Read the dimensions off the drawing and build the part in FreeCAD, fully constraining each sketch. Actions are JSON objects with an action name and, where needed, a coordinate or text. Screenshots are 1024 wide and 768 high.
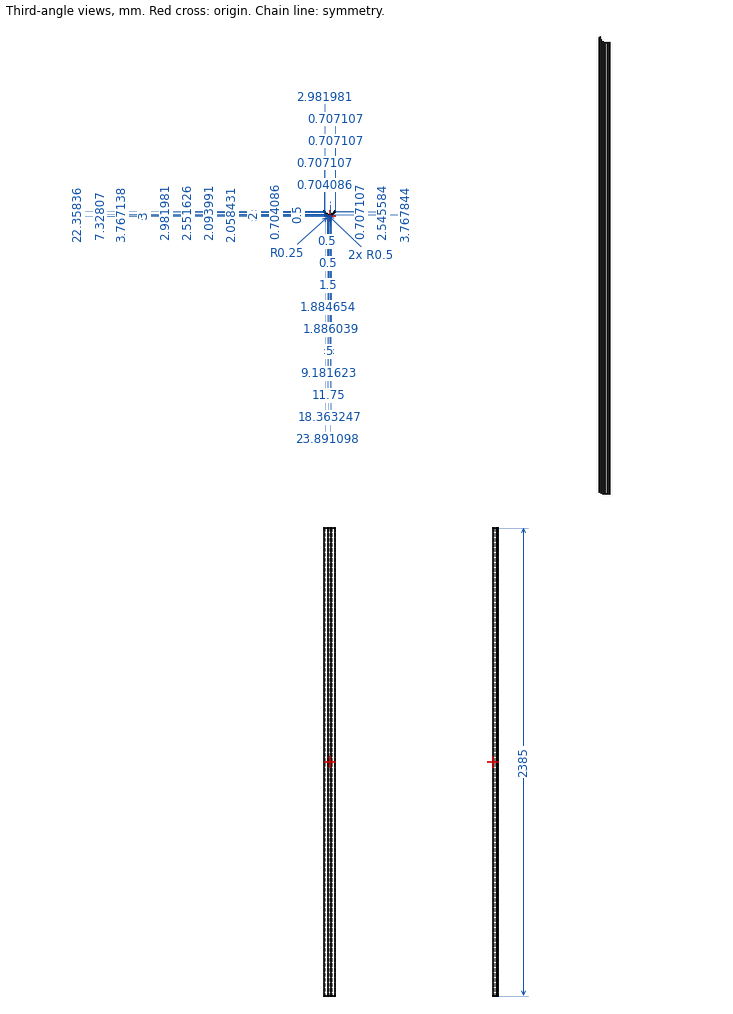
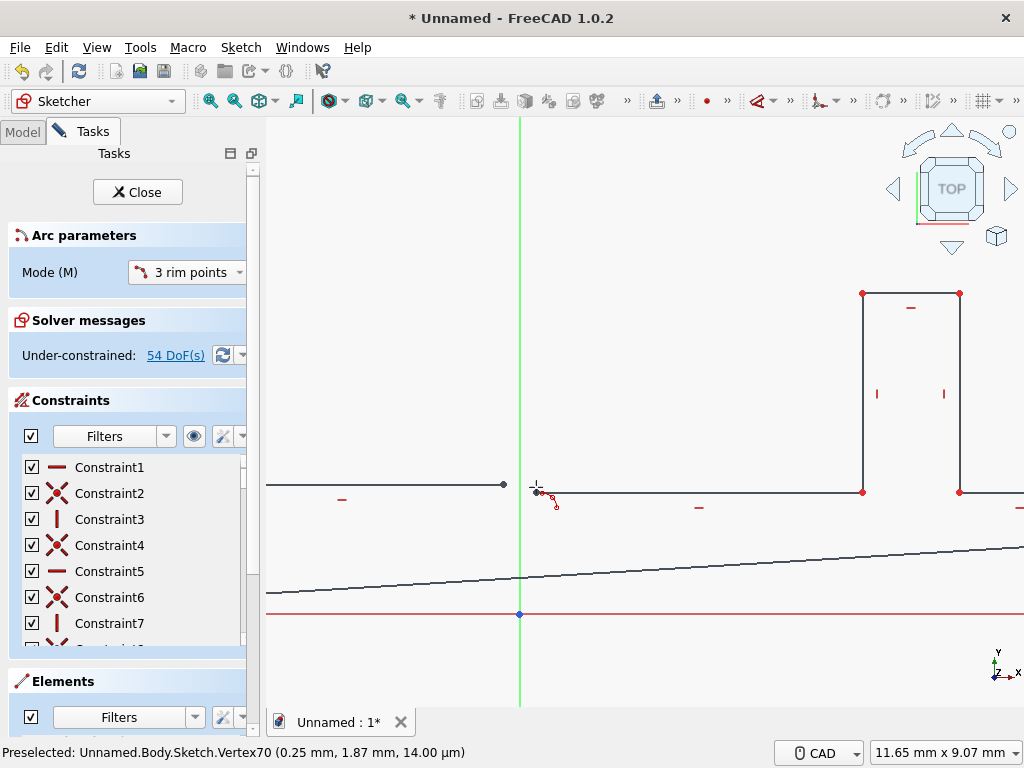
{"action": "scroll", "coordinate": [584, 477], "scroll_direction": "down", "scroll_amount": 11}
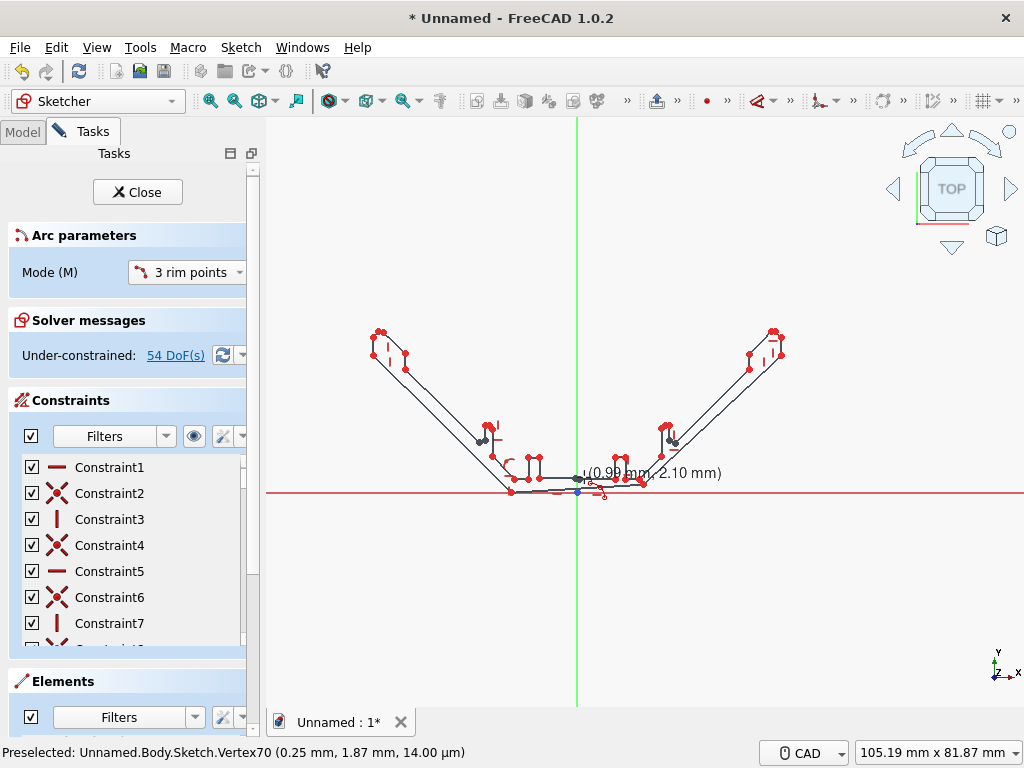
{"action": "scroll", "coordinate": [485, 440], "scroll_direction": "up", "scroll_amount": 5}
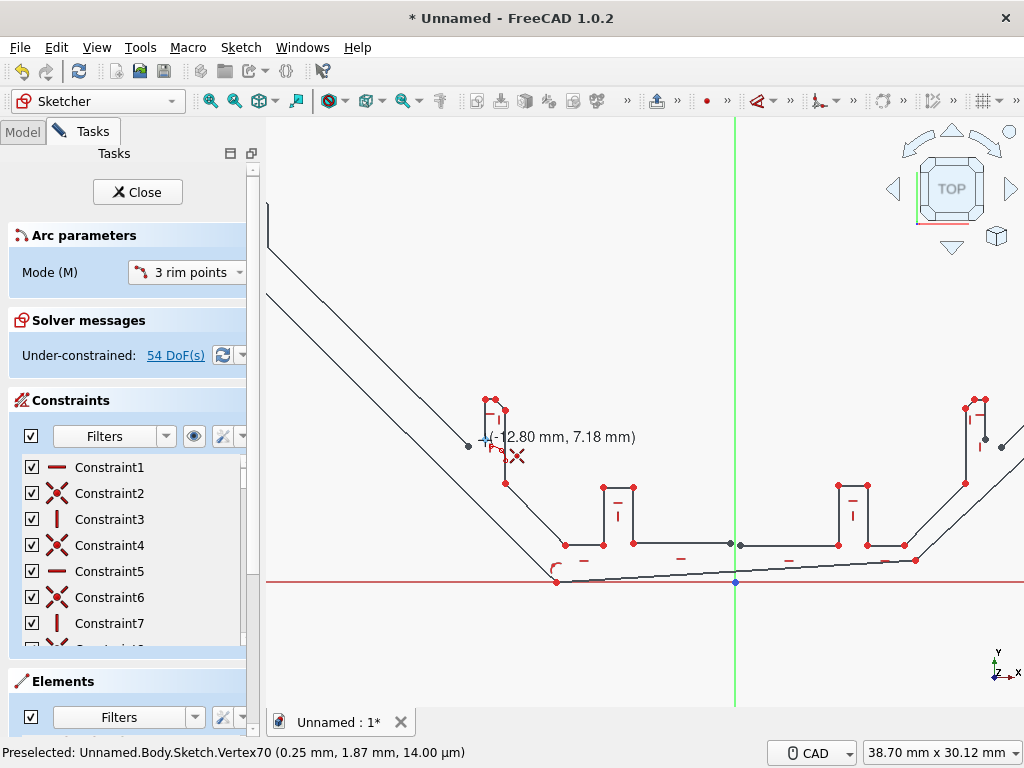
{"action": "left_click", "coordinate": [485, 440]}
{"action": "left_click", "coordinate": [469, 446]}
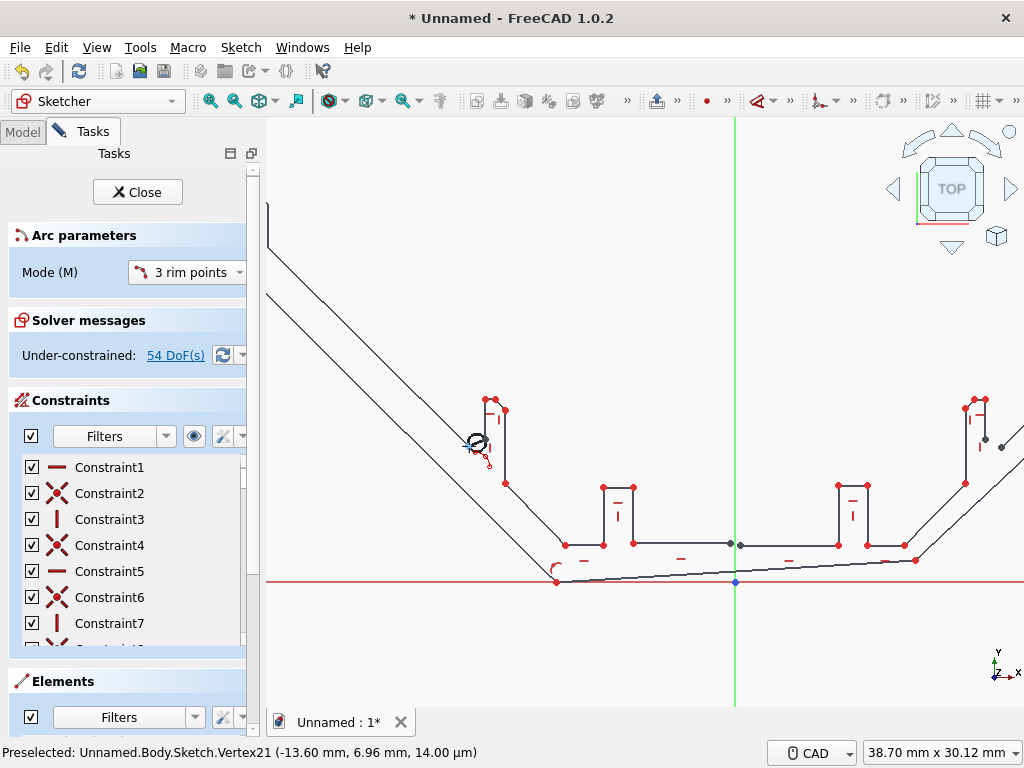
{"action": "scroll", "coordinate": [479, 448], "scroll_direction": "up", "scroll_amount": 5}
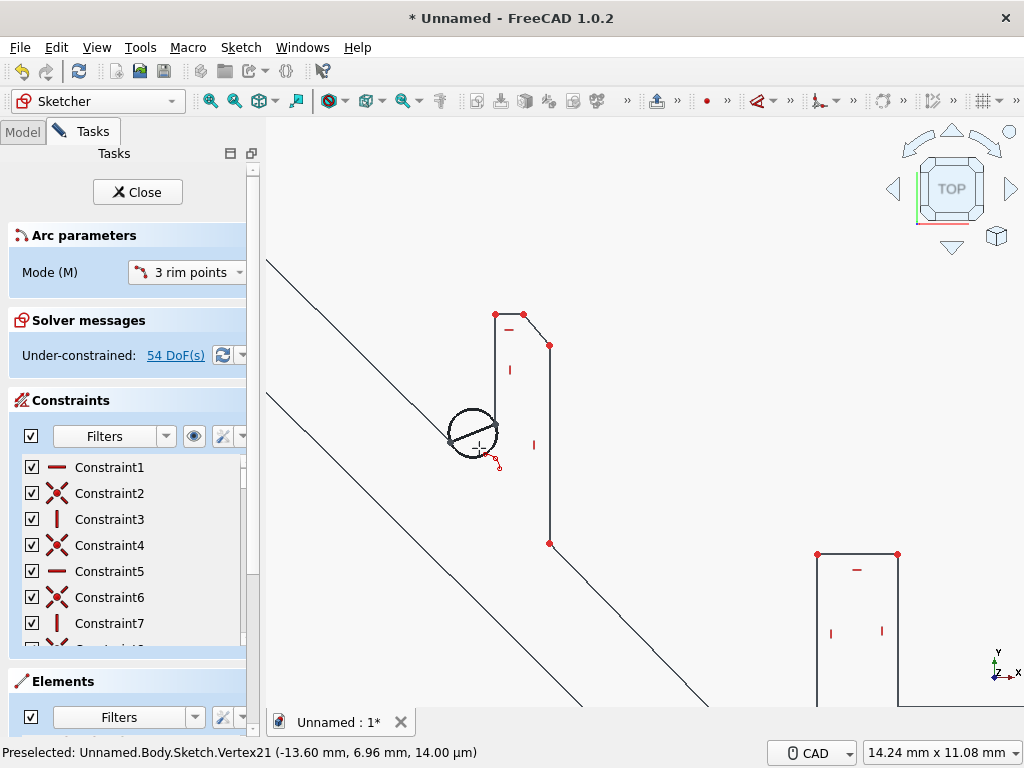
{"action": "left_click", "coordinate": [480, 447]}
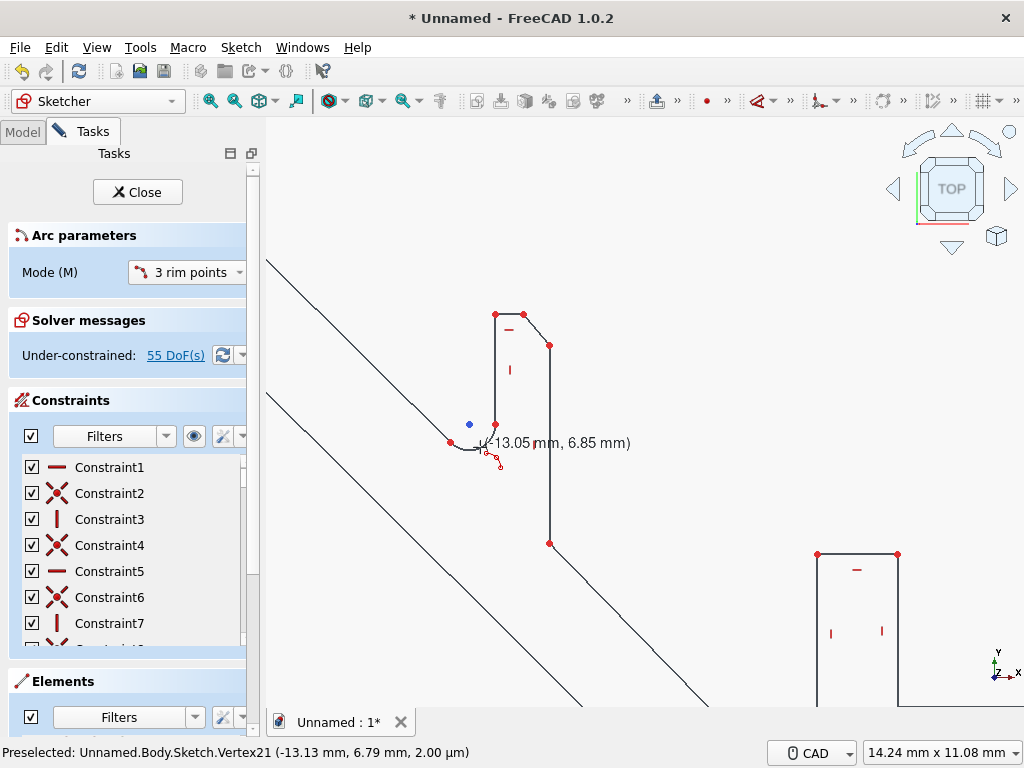
{"action": "scroll", "coordinate": [483, 442], "scroll_direction": "down", "scroll_amount": 10}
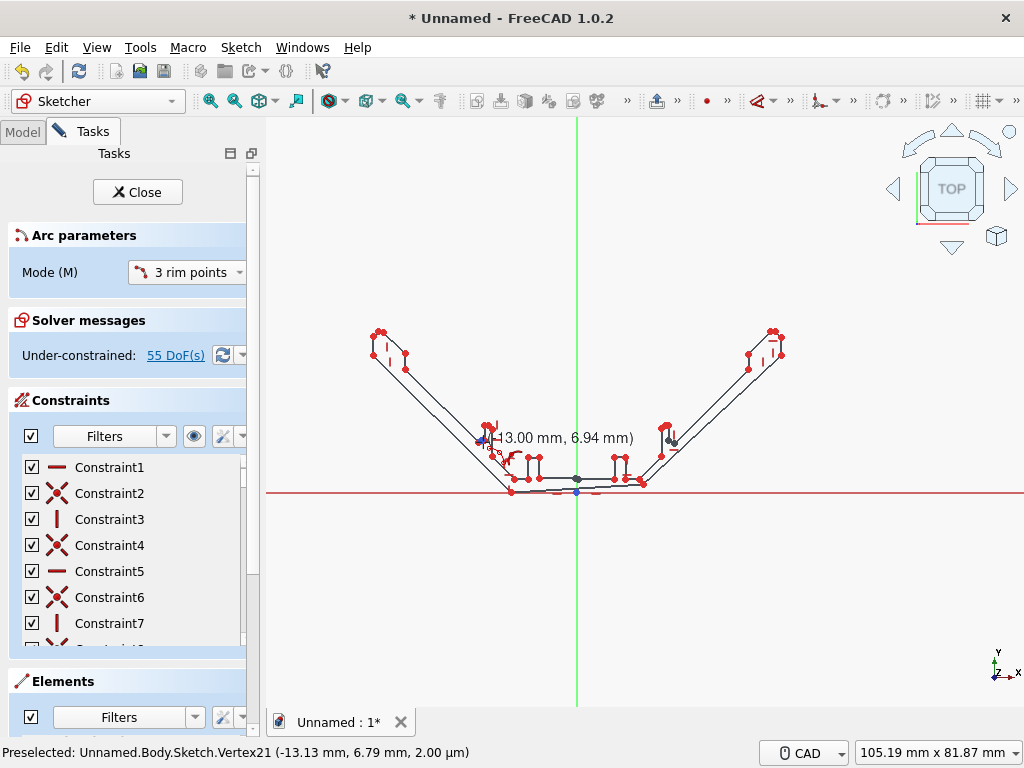
{"action": "scroll", "coordinate": [675, 442], "scroll_direction": "up", "scroll_amount": 5}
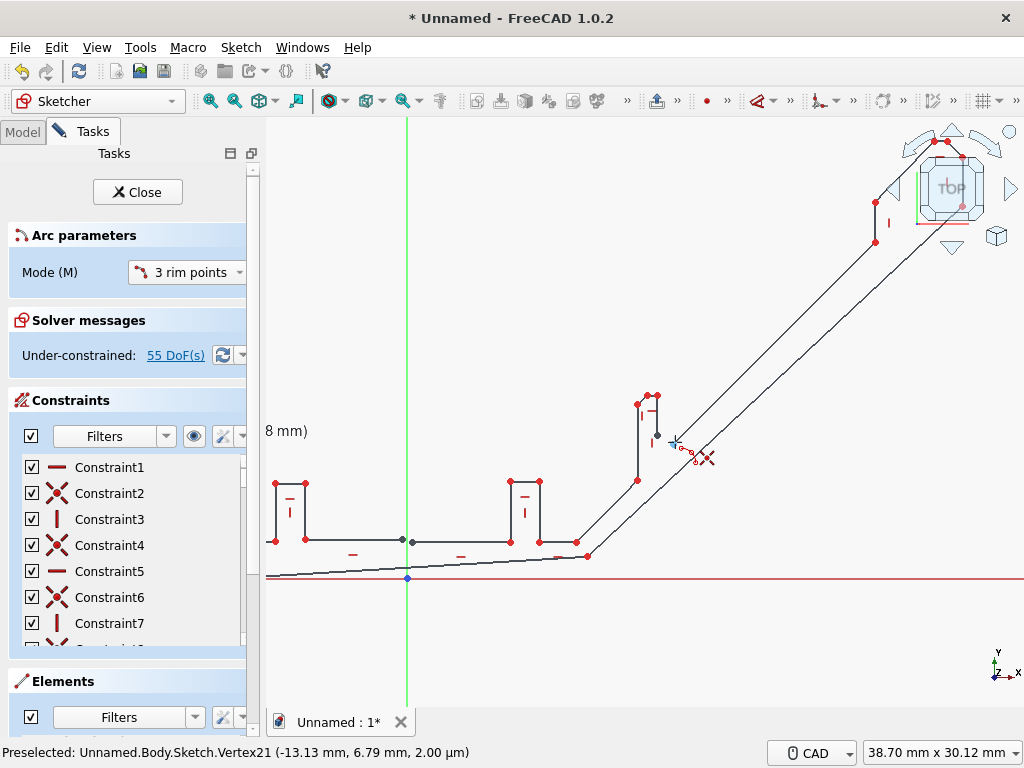
{"action": "left_click", "coordinate": [674, 444]}
{"action": "left_click", "coordinate": [657, 436]}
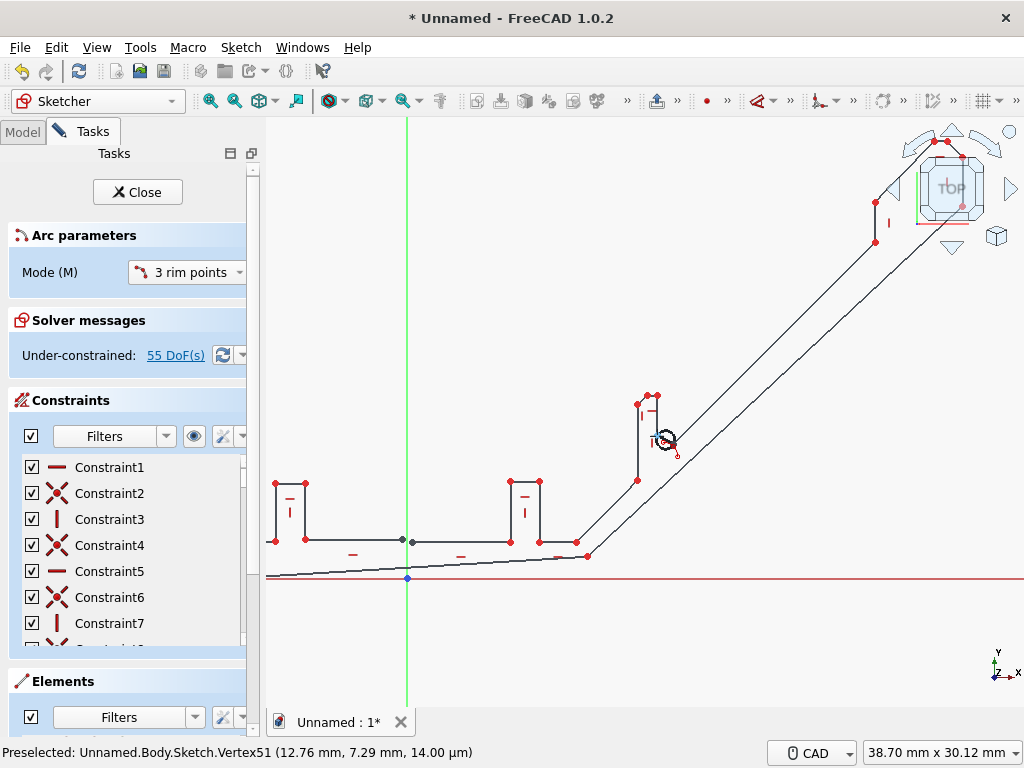
{"action": "scroll", "coordinate": [663, 444], "scroll_direction": "up", "scroll_amount": 5}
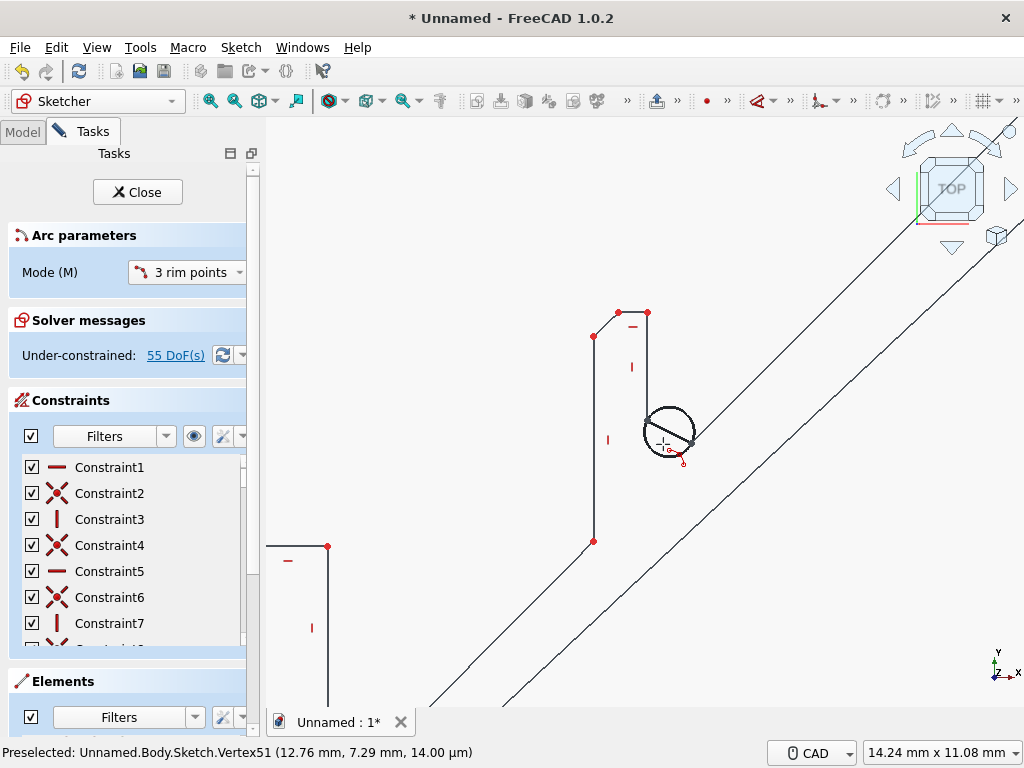
{"action": "left_click", "coordinate": [663, 443]}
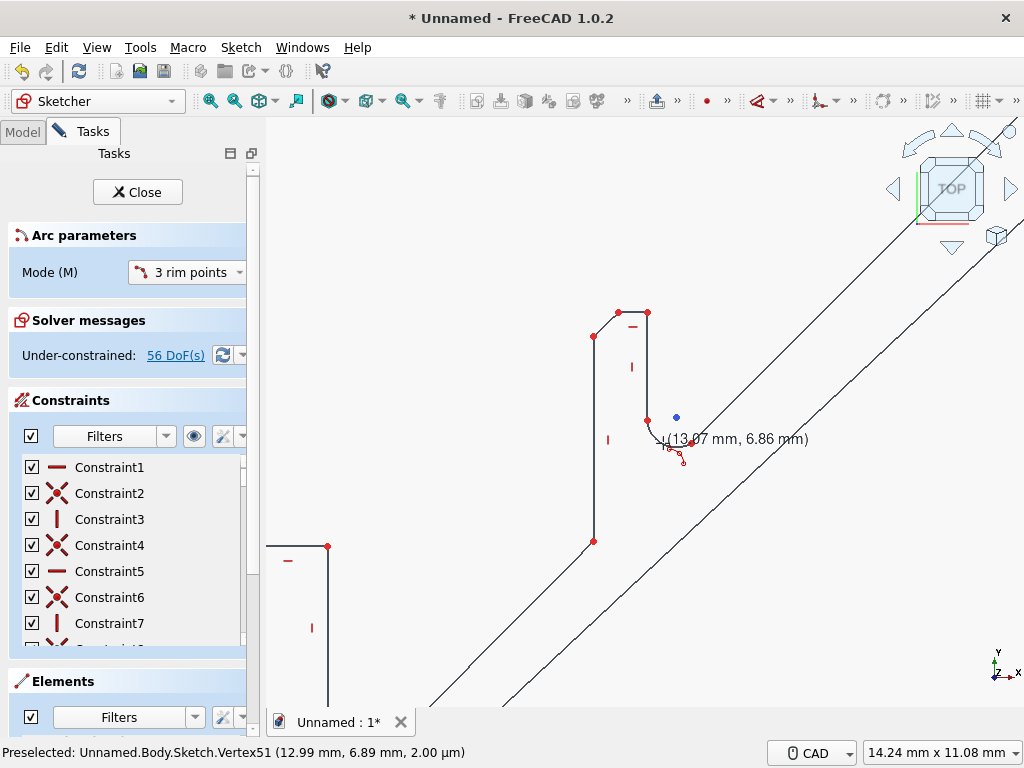
{"action": "scroll", "coordinate": [672, 443], "scroll_direction": "down", "scroll_amount": 10}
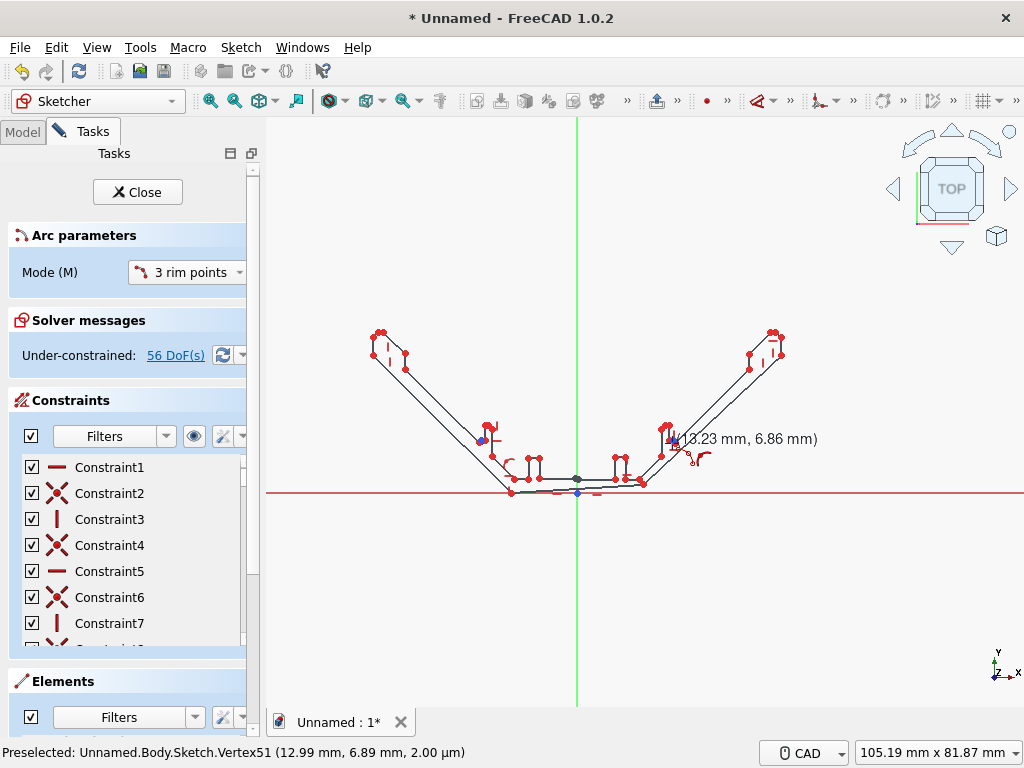
{"action": "scroll", "coordinate": [579, 479], "scroll_direction": "up", "scroll_amount": 11}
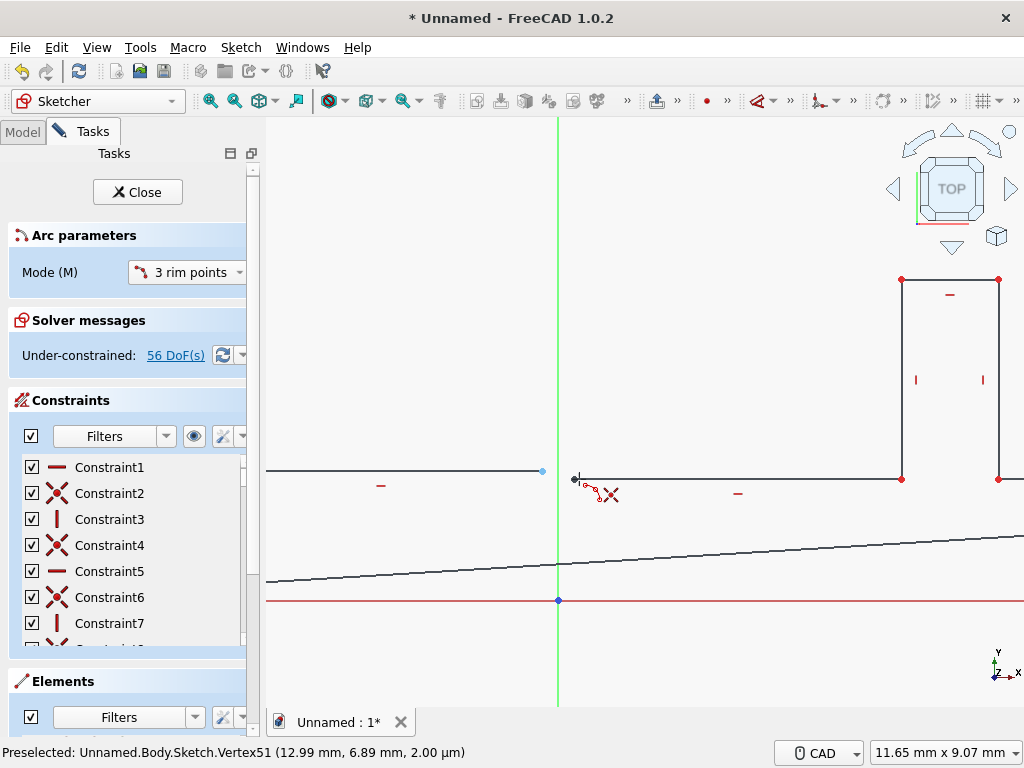
{"action": "left_click", "coordinate": [575, 479]}
{"action": "left_click", "coordinate": [542, 471]}